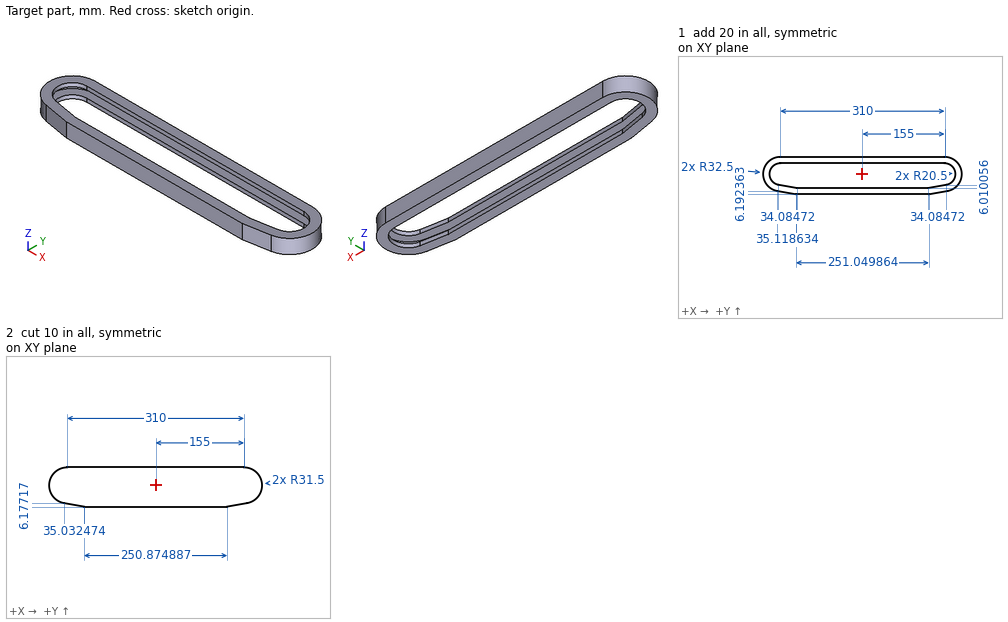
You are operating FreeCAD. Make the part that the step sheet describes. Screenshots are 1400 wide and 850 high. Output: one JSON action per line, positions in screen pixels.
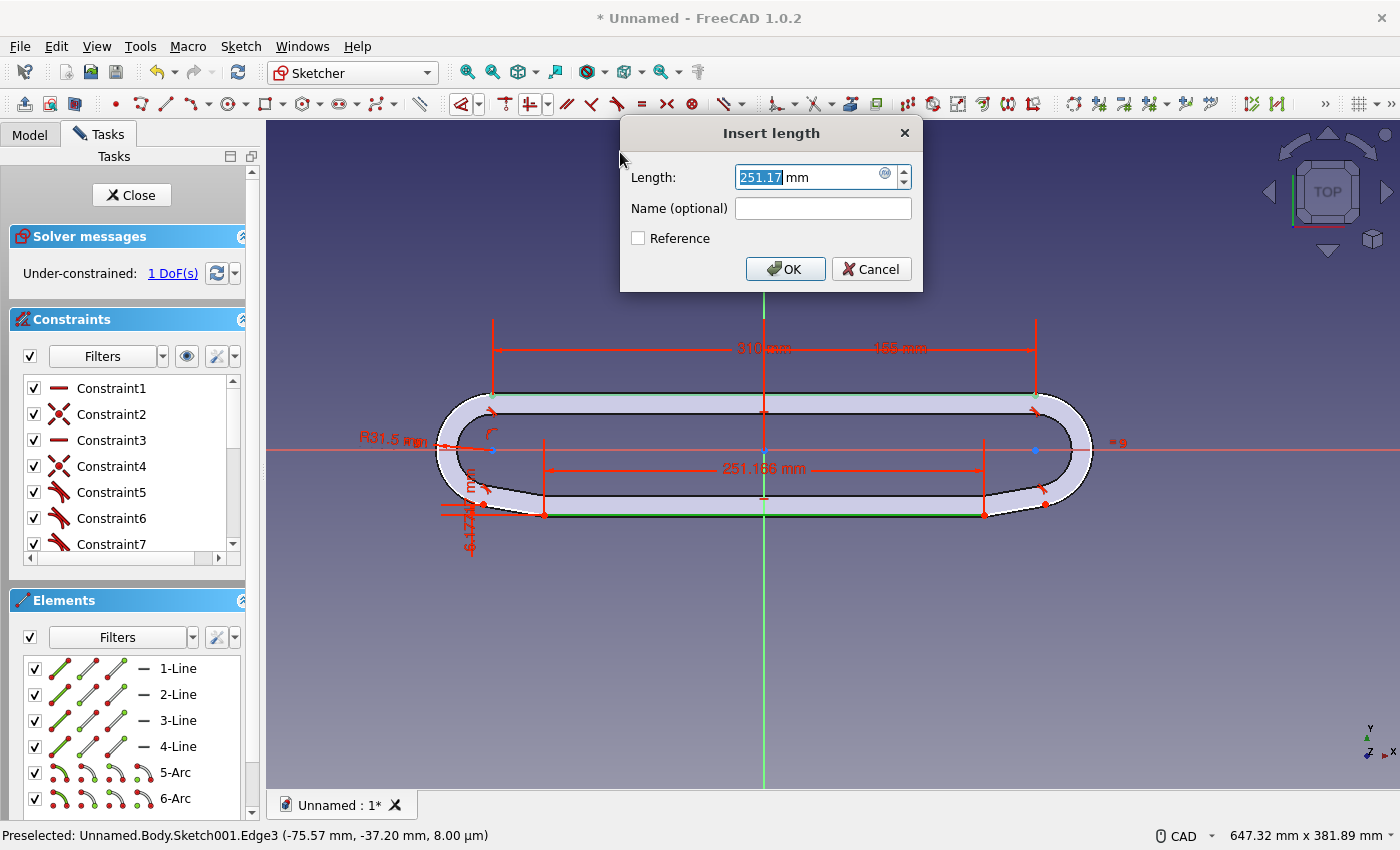
{"action": "type", "text": "250.874887"}
{"action": "key", "text": "Return"}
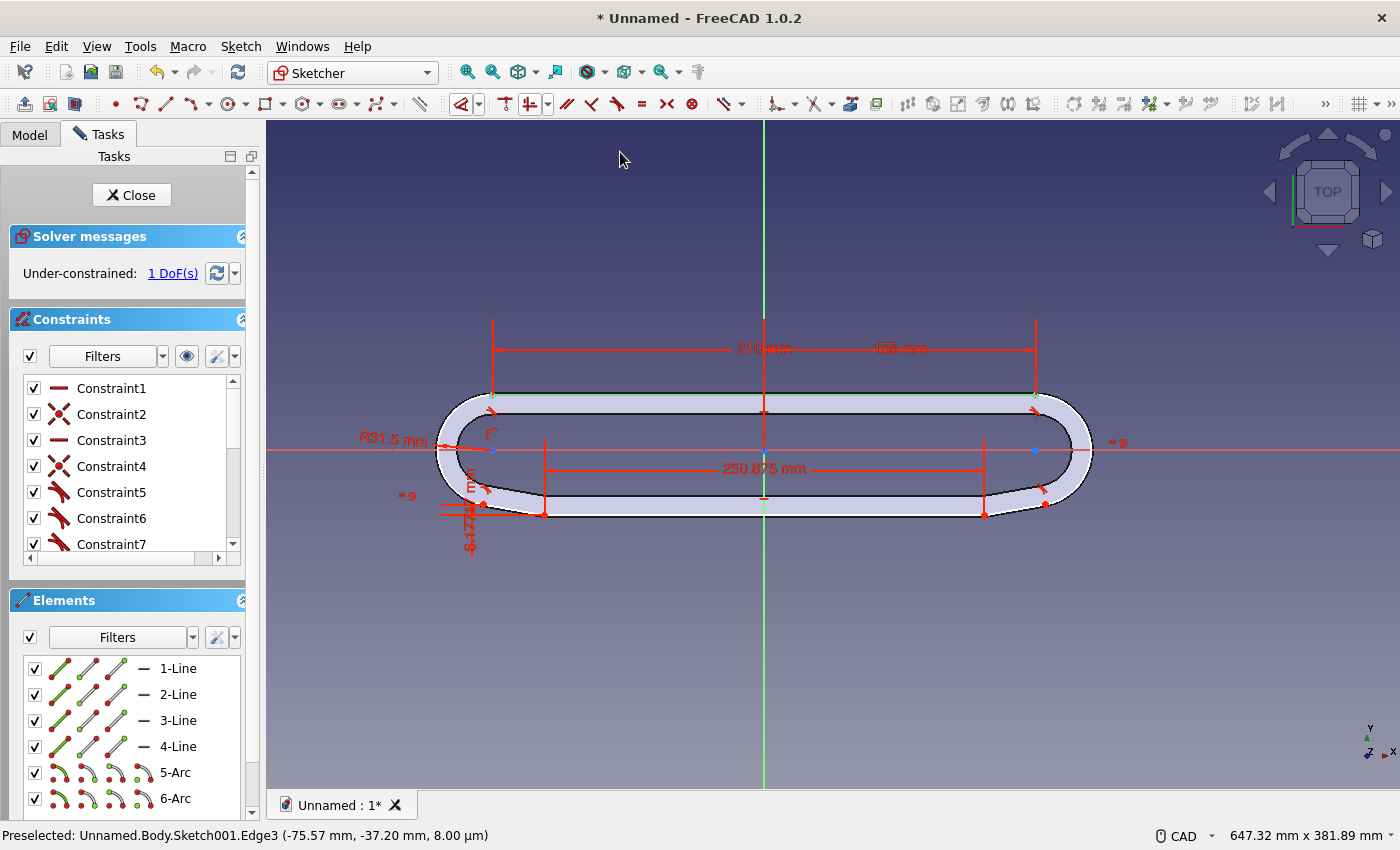
{"action": "left_click", "coordinate": [502, 508]}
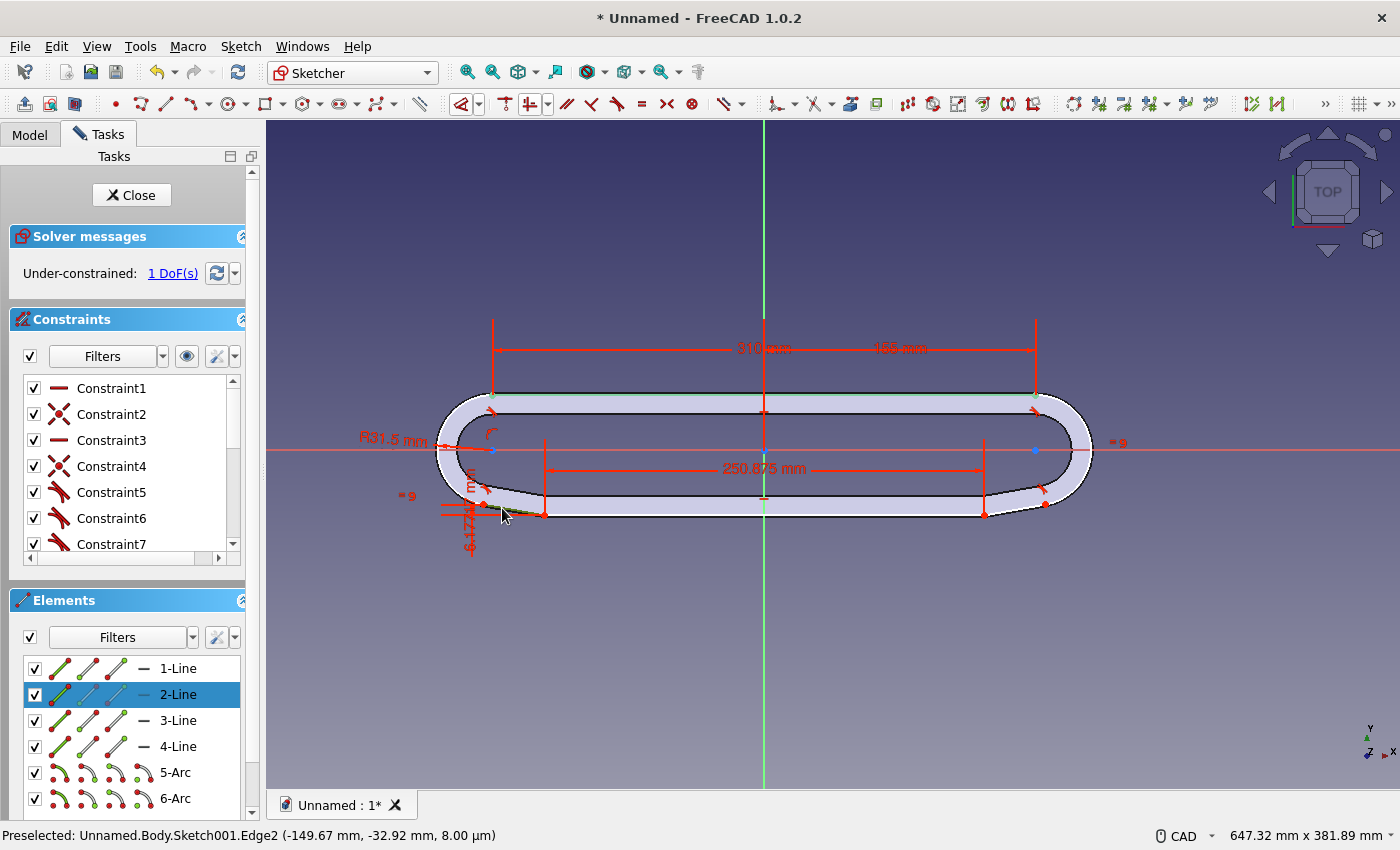
{"action": "key", "text": "l"}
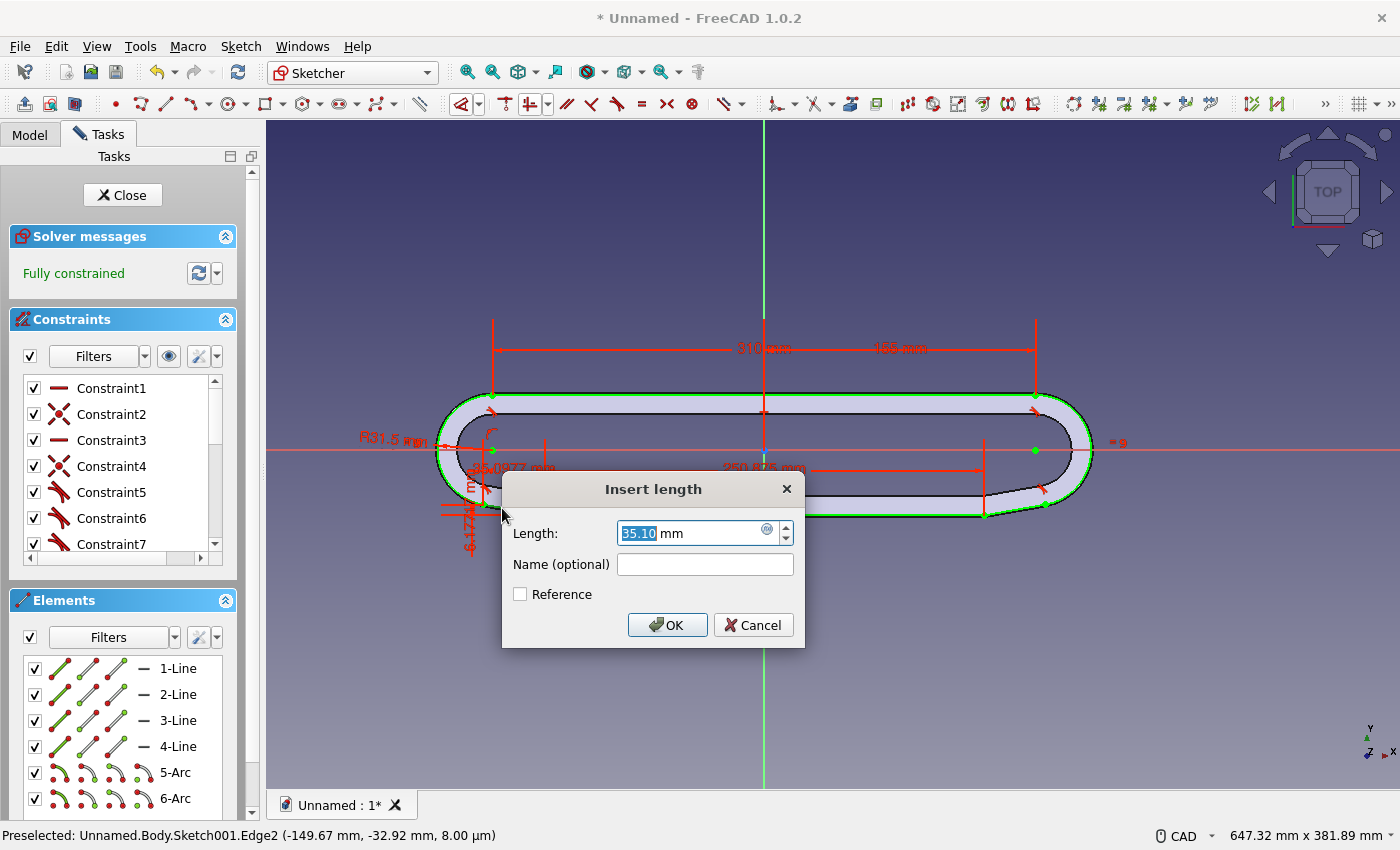
{"action": "type", "text": "35.032474"}
{"action": "key", "text": "Return"}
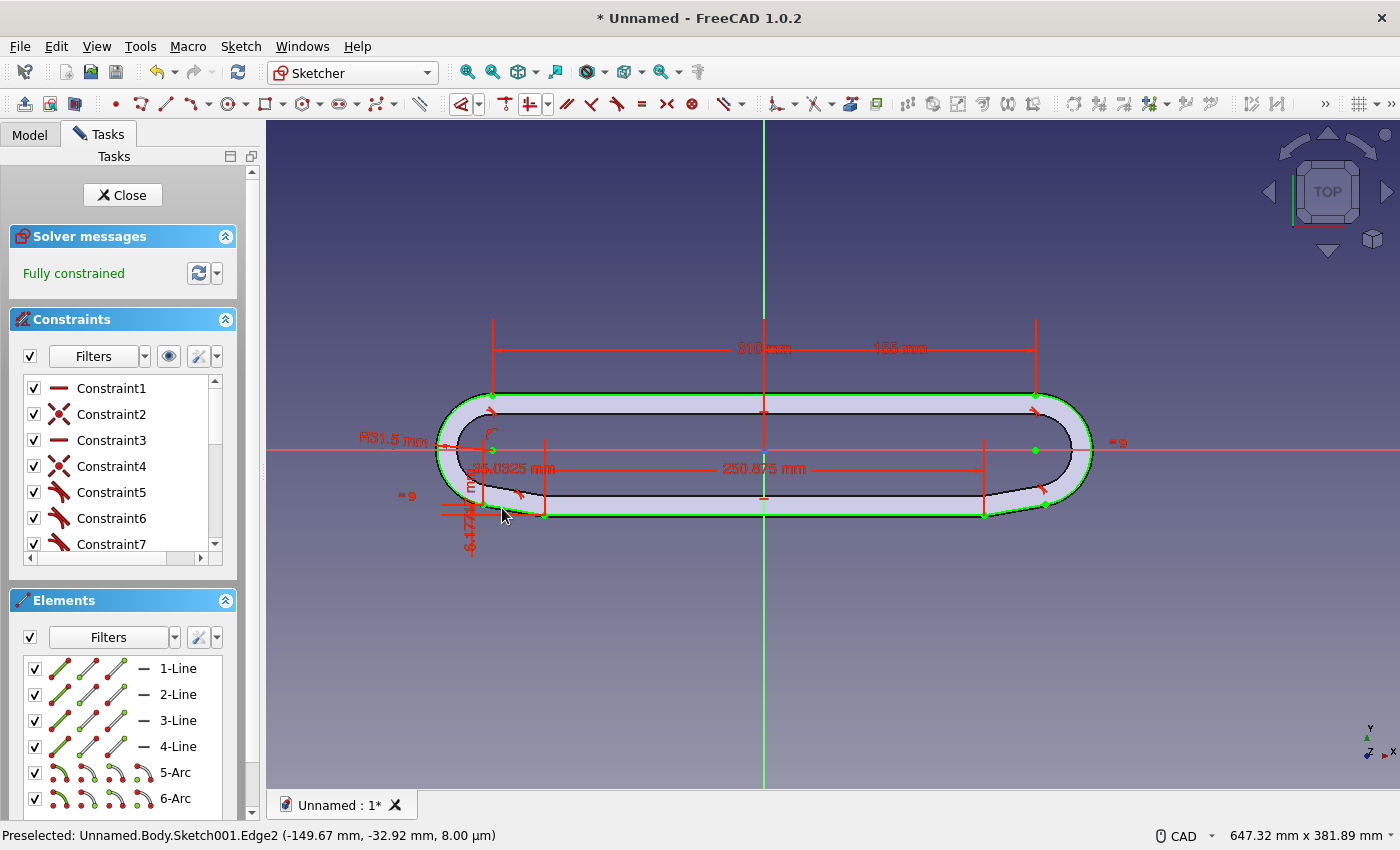
{"action": "left_click", "coordinate": [123, 195]}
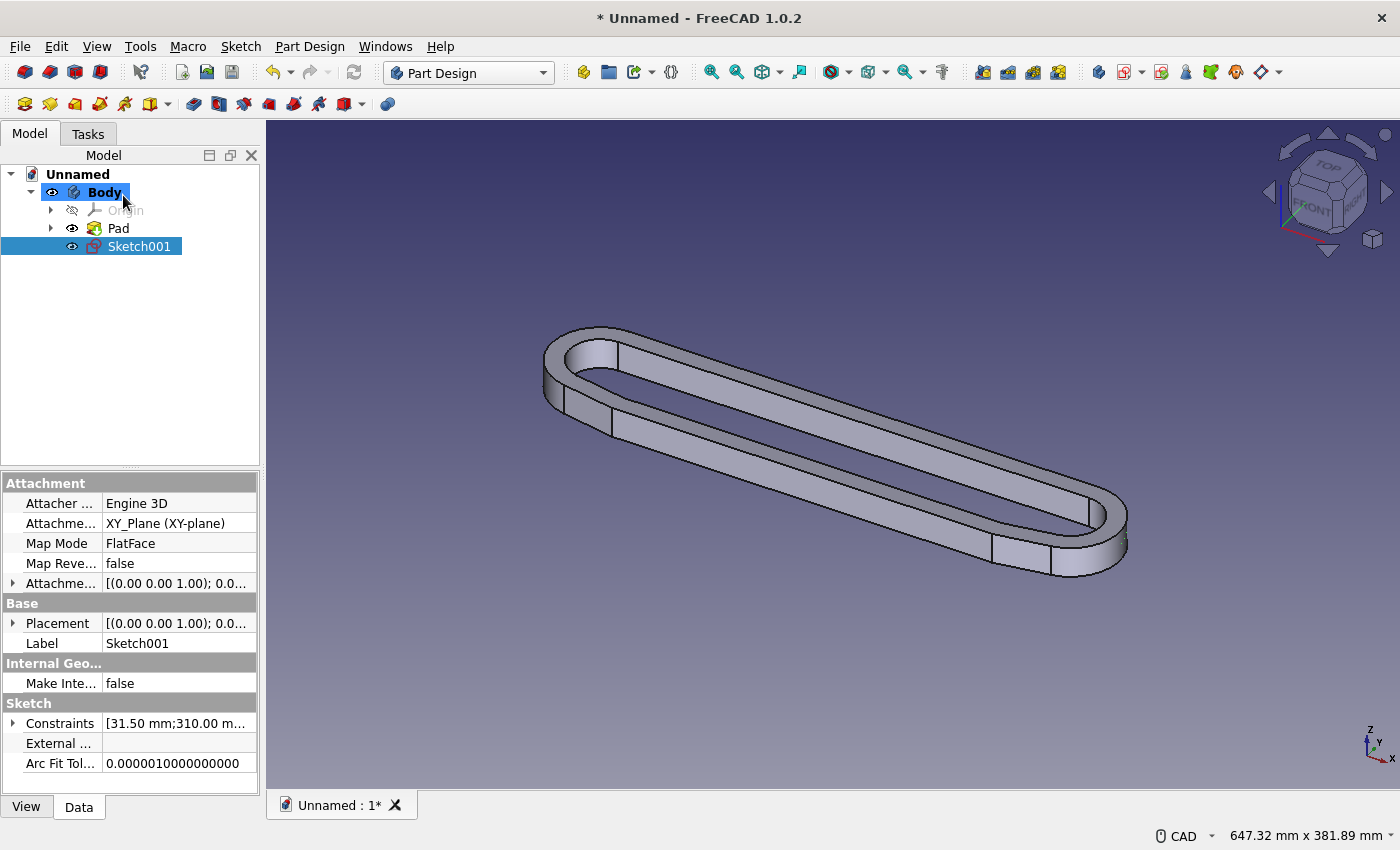
{"action": "left_click", "coordinate": [194, 104]}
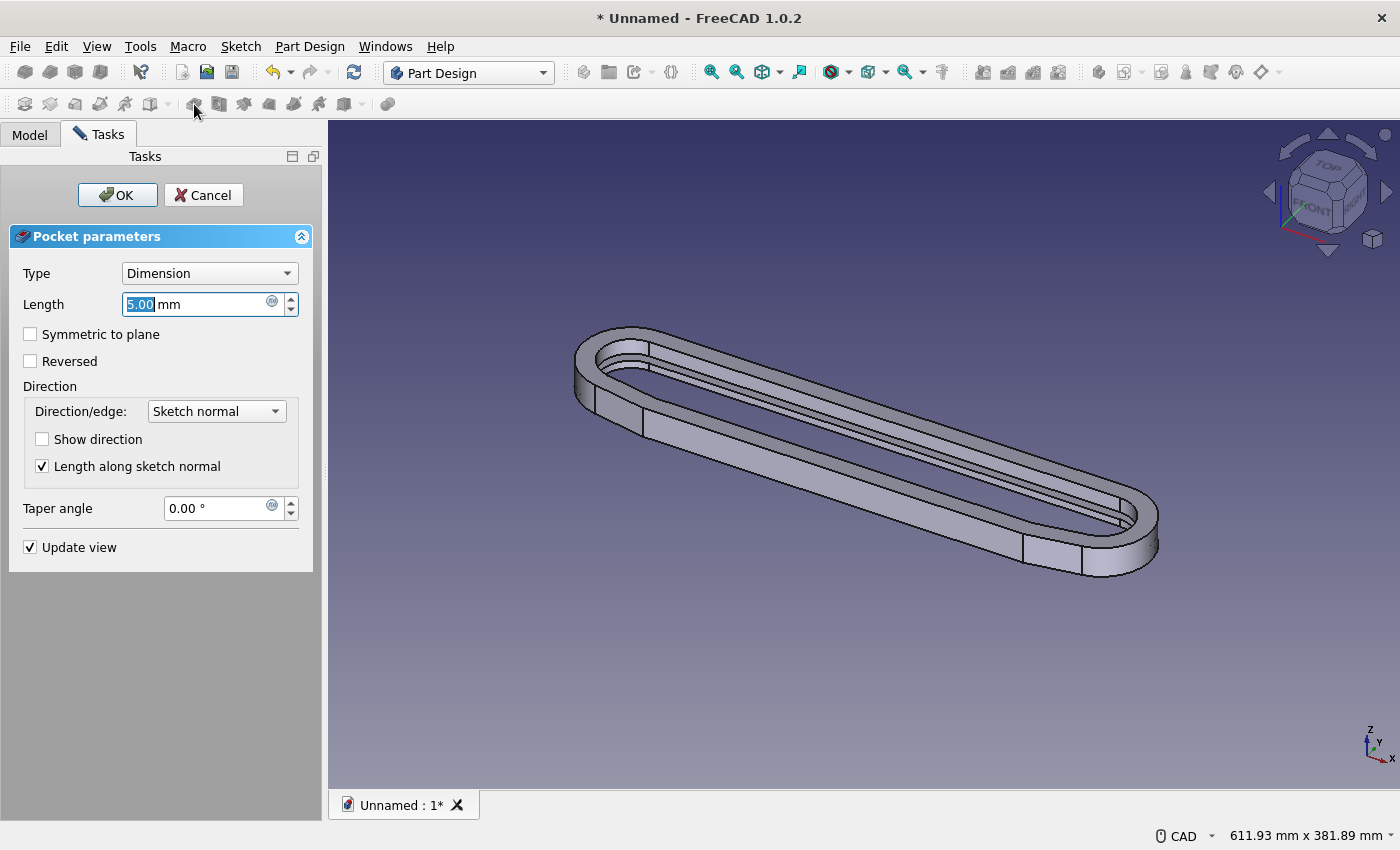
{"action": "type", "text": "10"}
{"action": "key", "text": "Tab"}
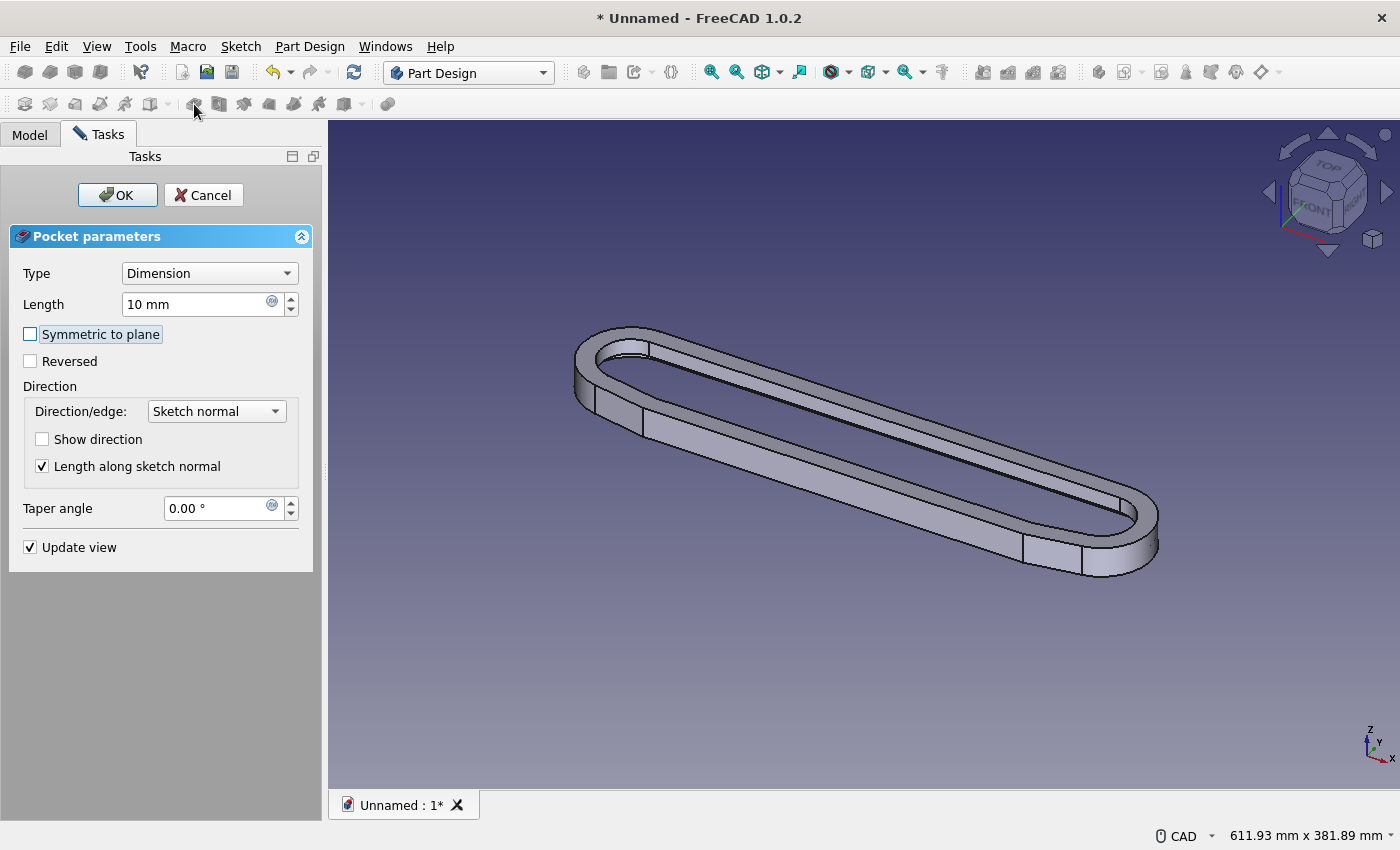
{"action": "left_click", "coordinate": [31, 334]}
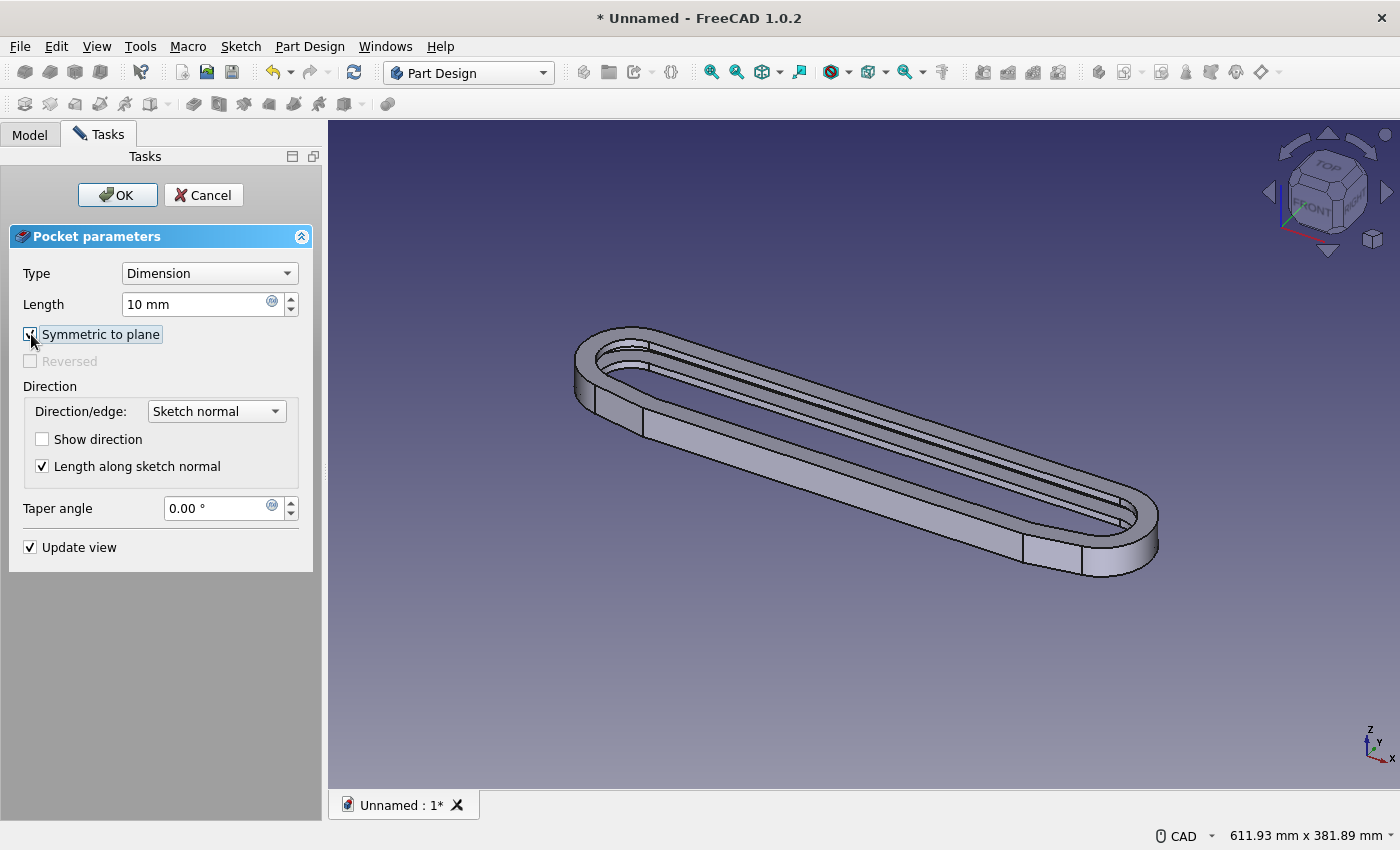
{"action": "left_click", "coordinate": [118, 195]}